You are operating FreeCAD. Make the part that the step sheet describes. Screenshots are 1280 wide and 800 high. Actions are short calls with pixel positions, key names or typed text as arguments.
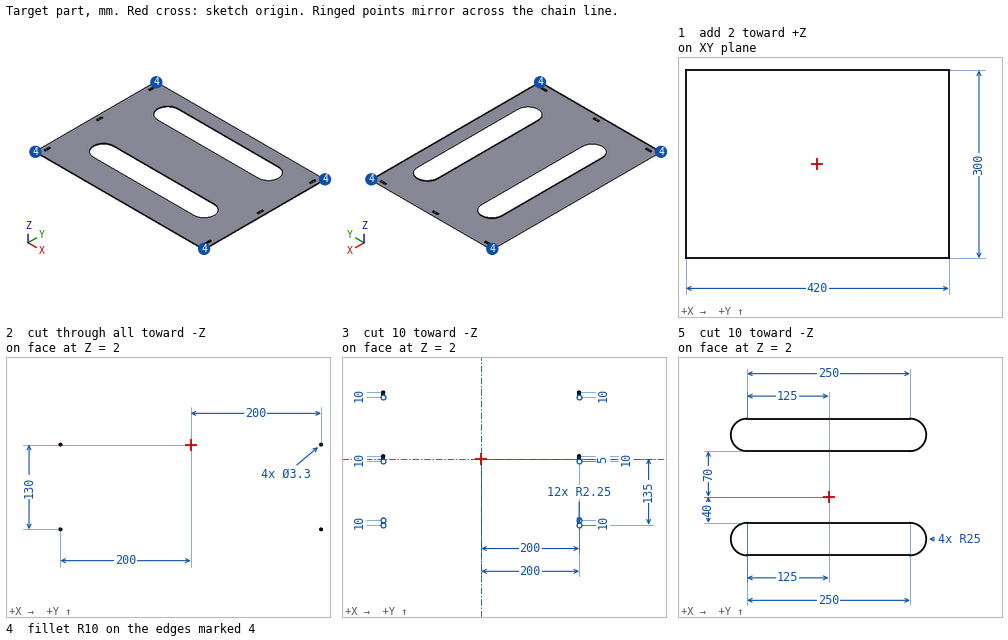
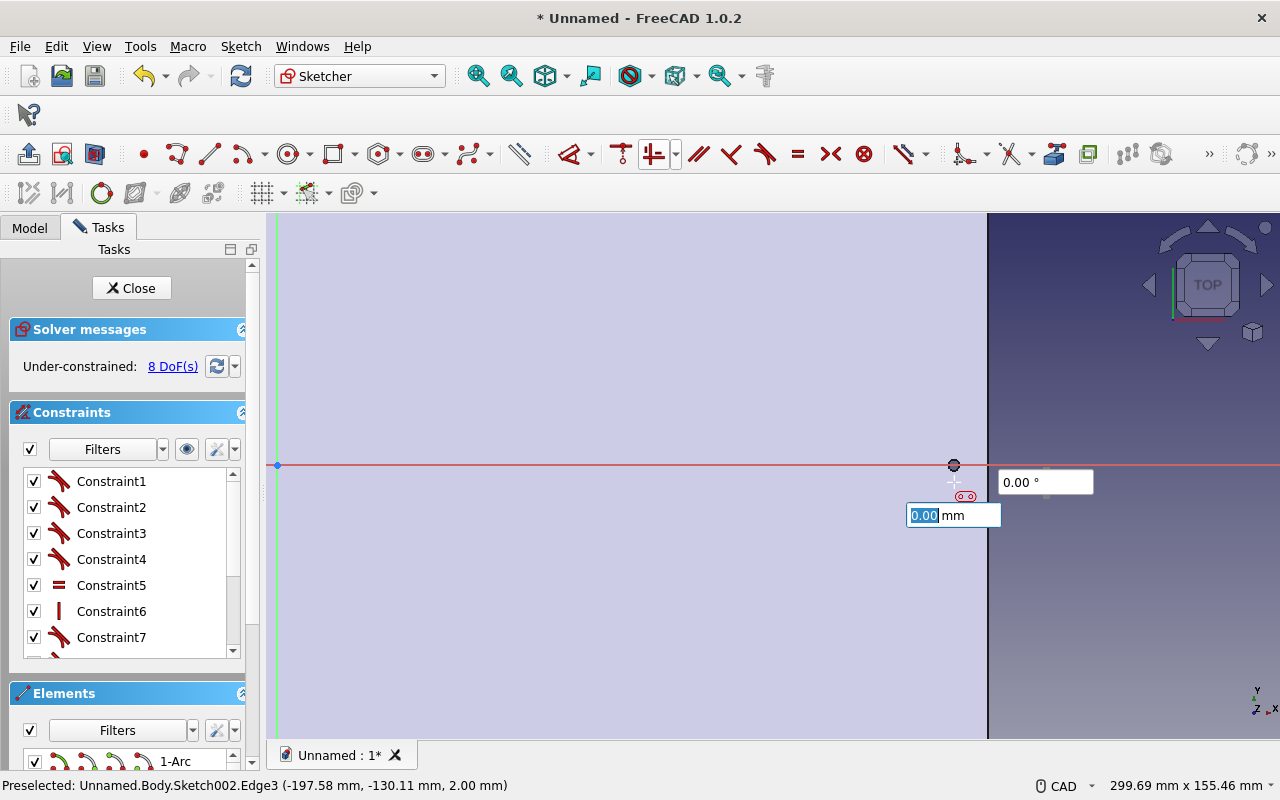
click(954, 448)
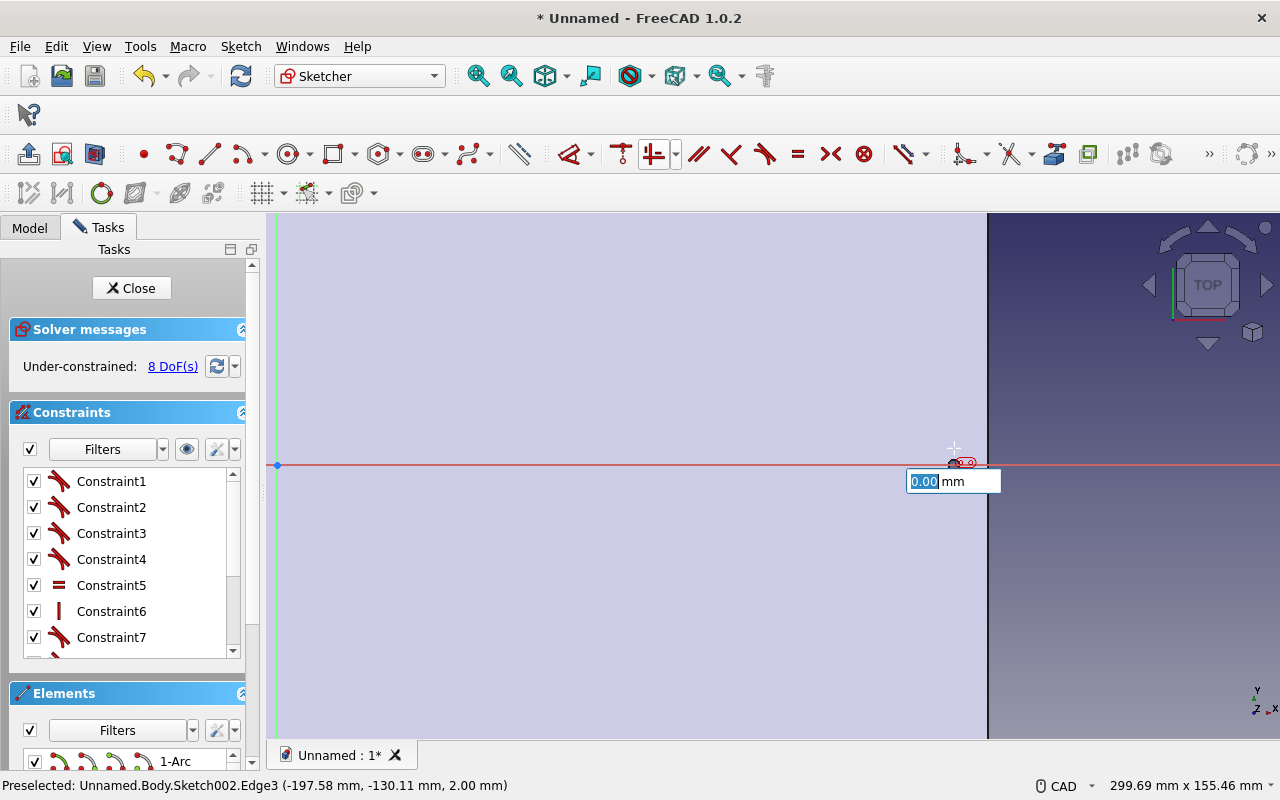
scroll(962, 470, up, 6)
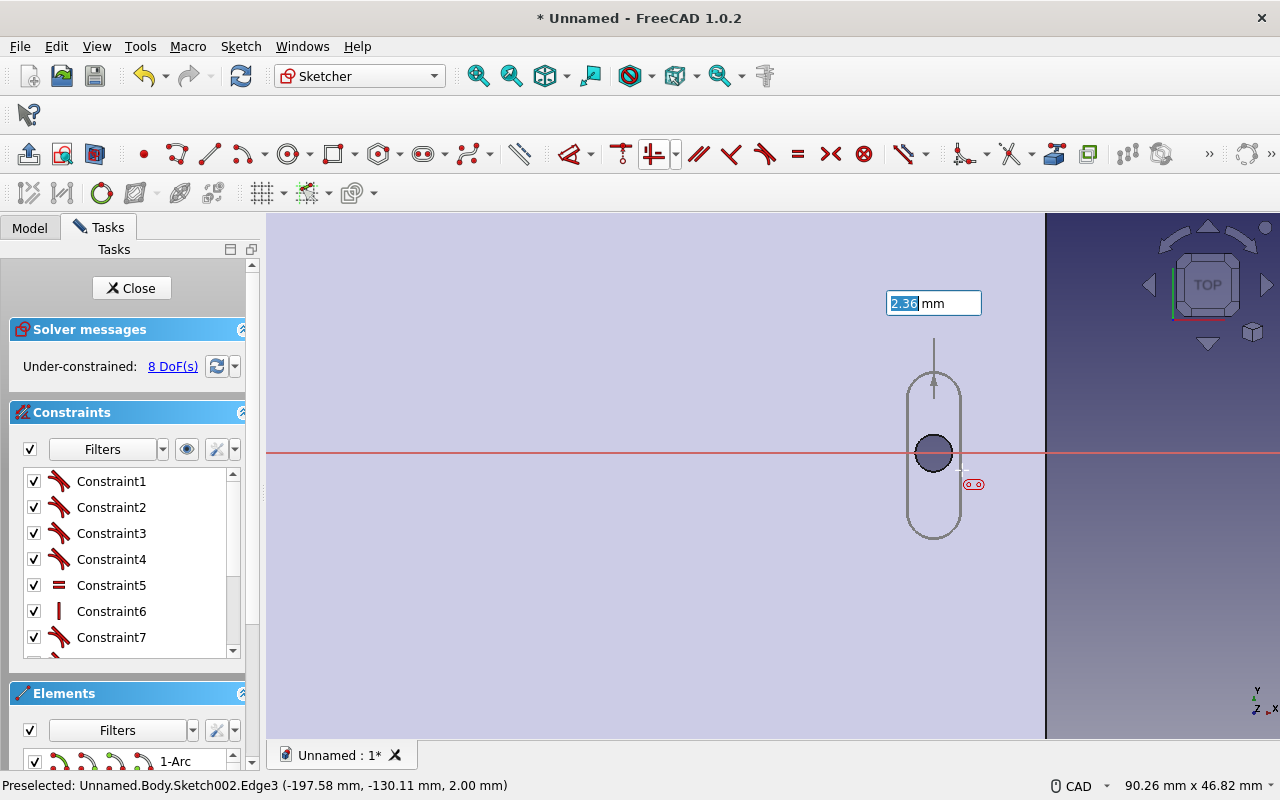
click(959, 470)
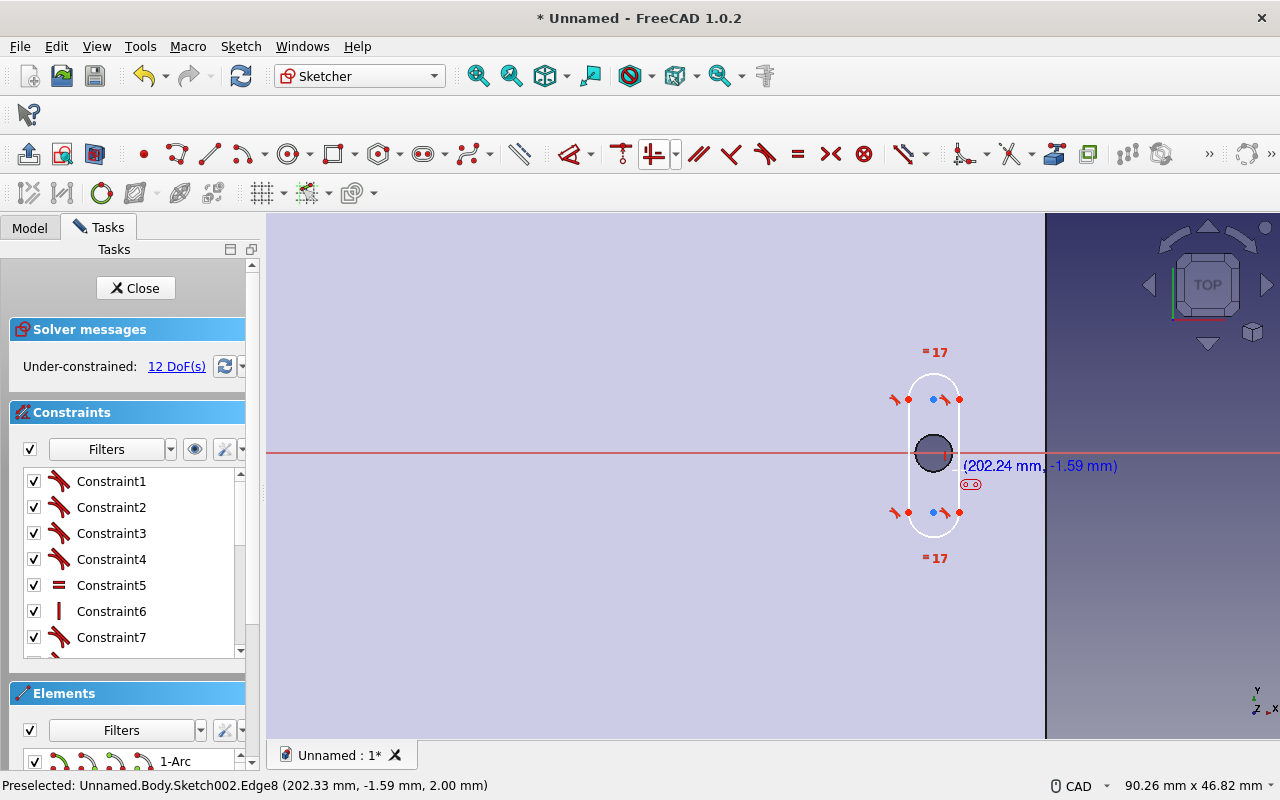
scroll(956, 479, down, 11)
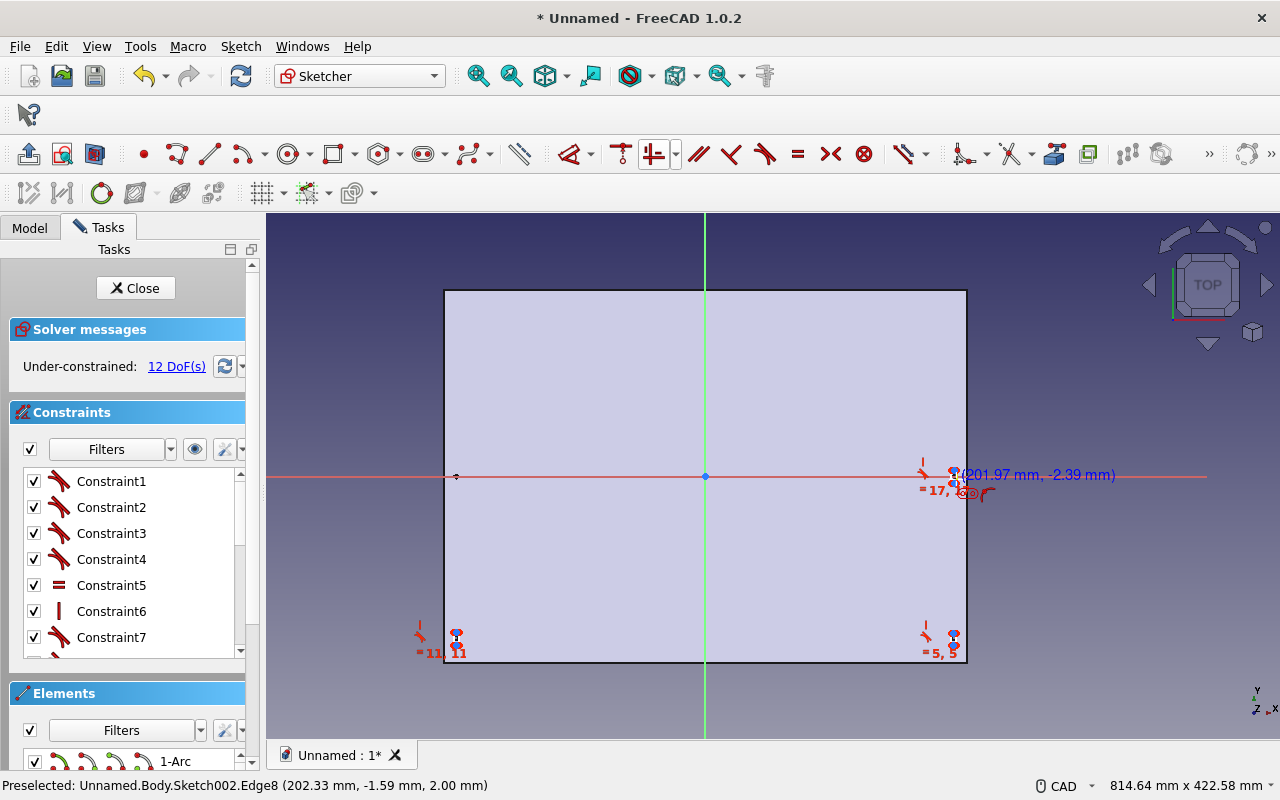
scroll(954, 321, up, 11)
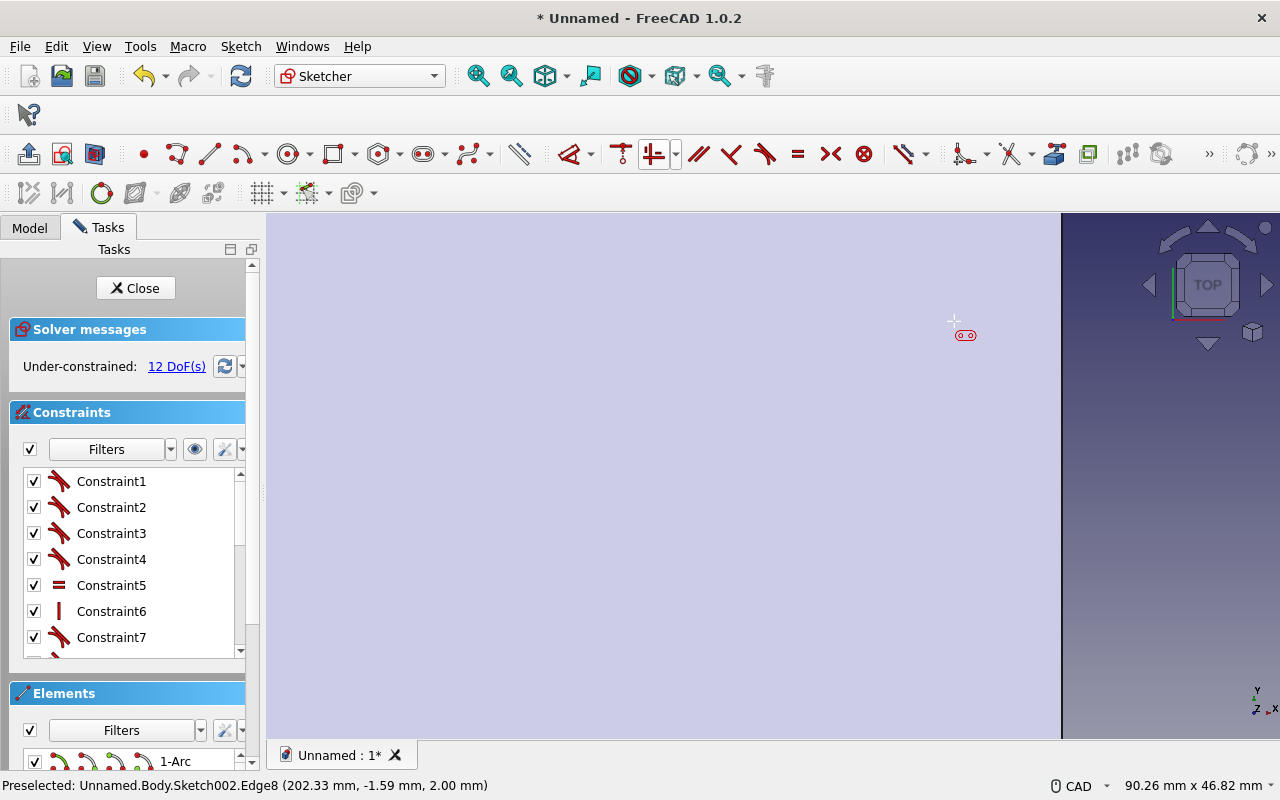
scroll(954, 321, down, 11)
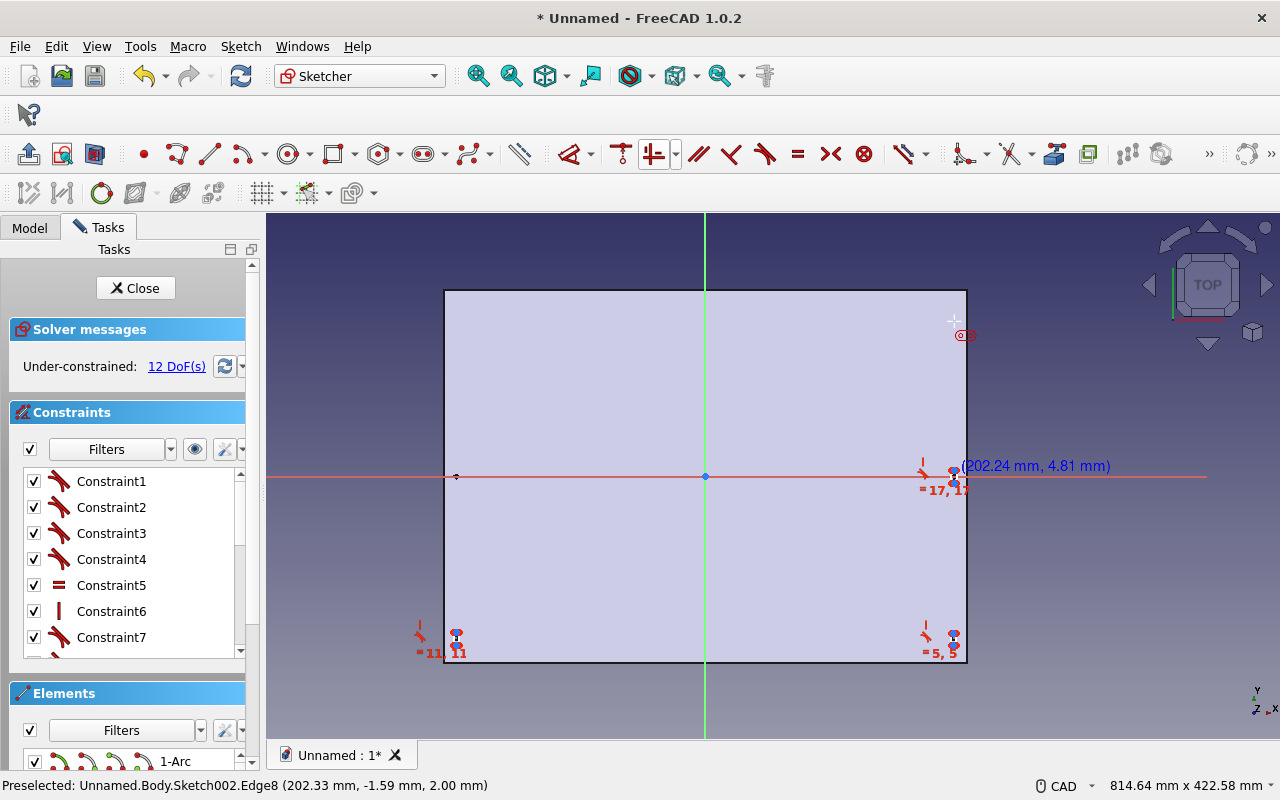
click(954, 321)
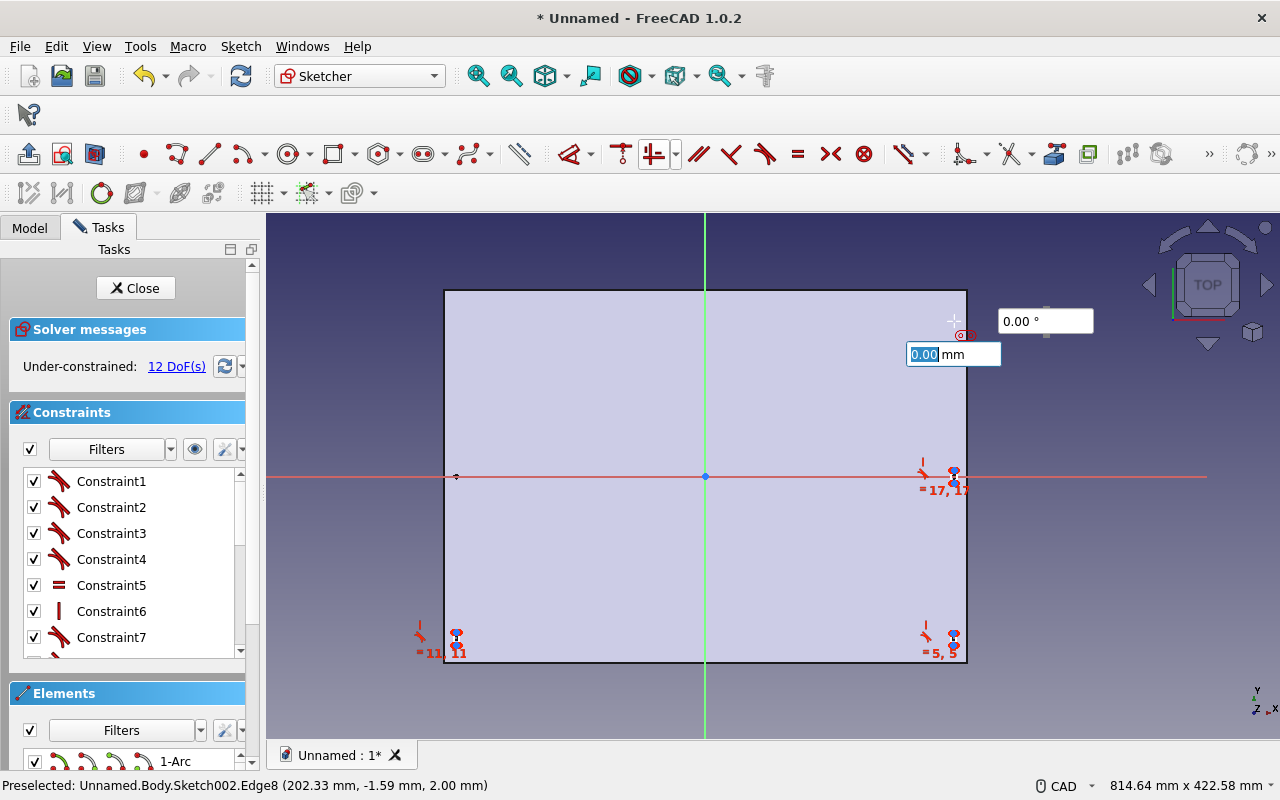
scroll(954, 309, up, 2)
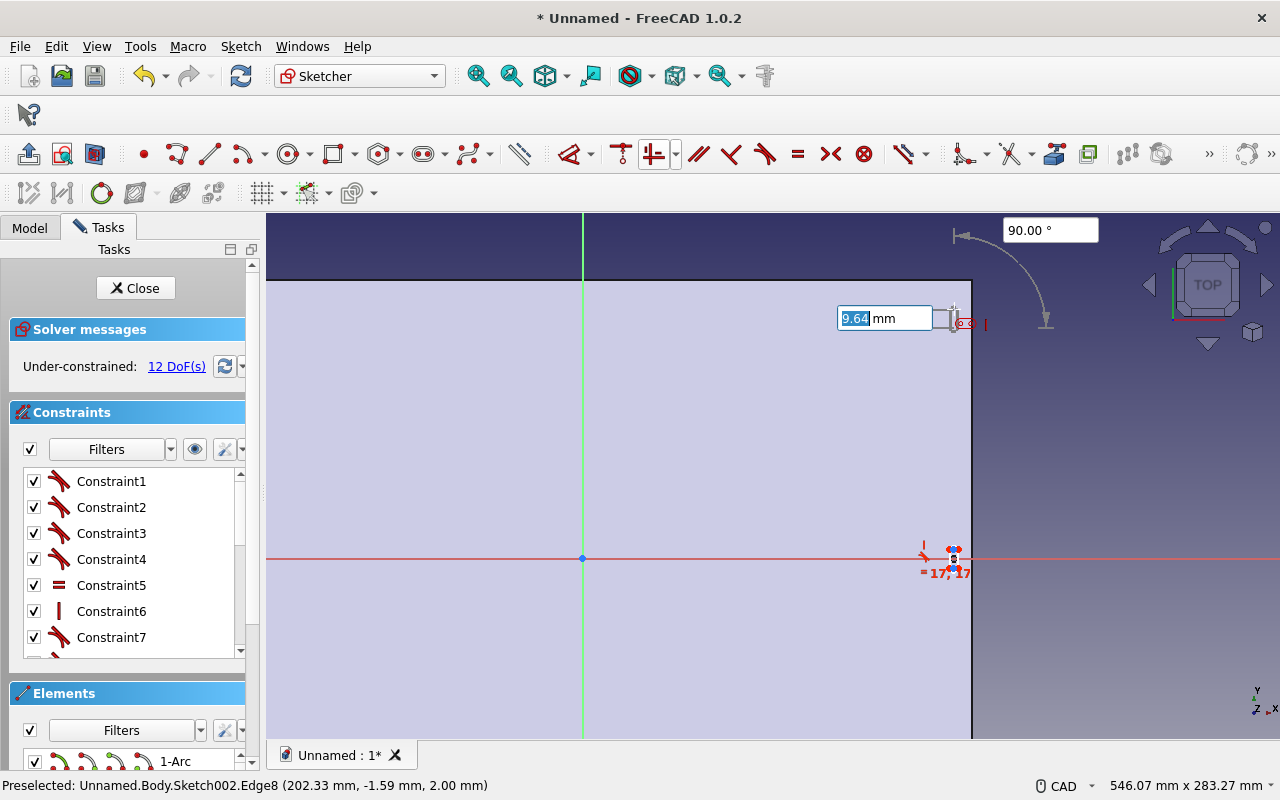
click(954, 308)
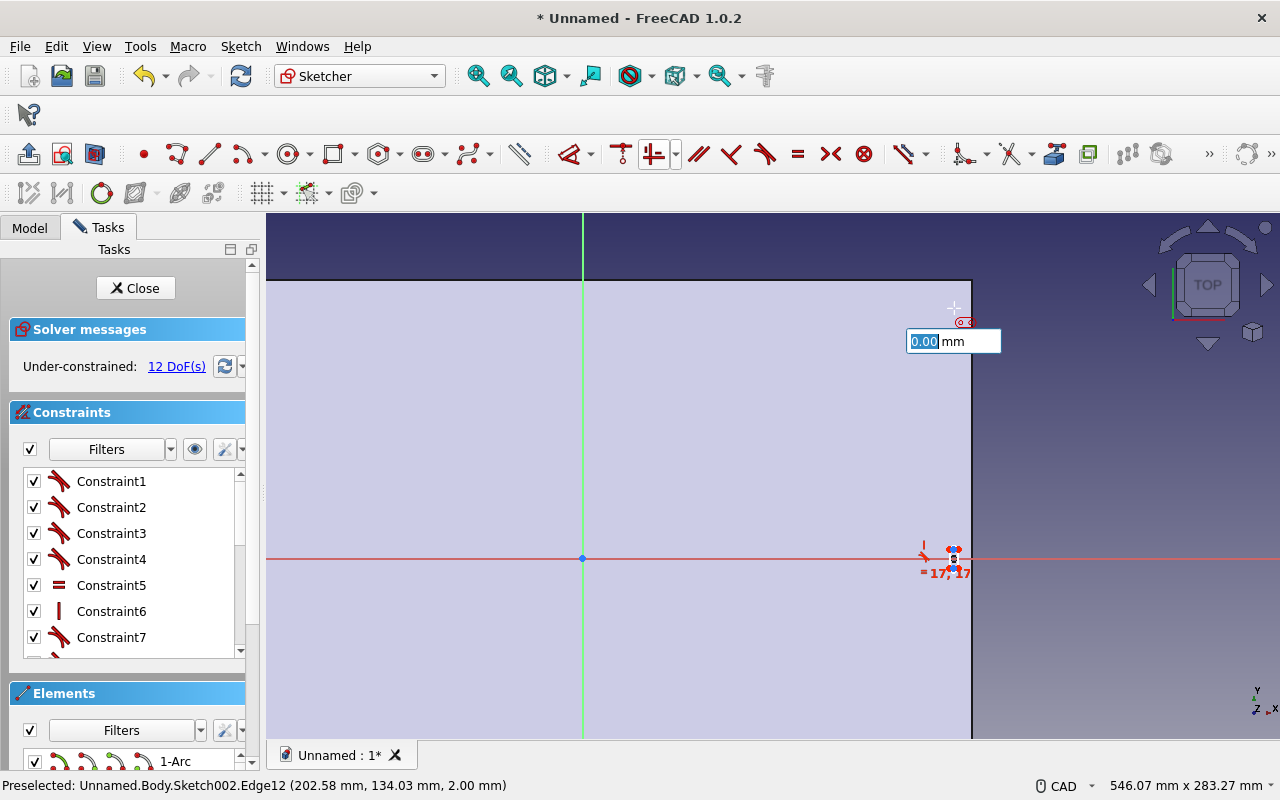
scroll(950, 318, up, 7)